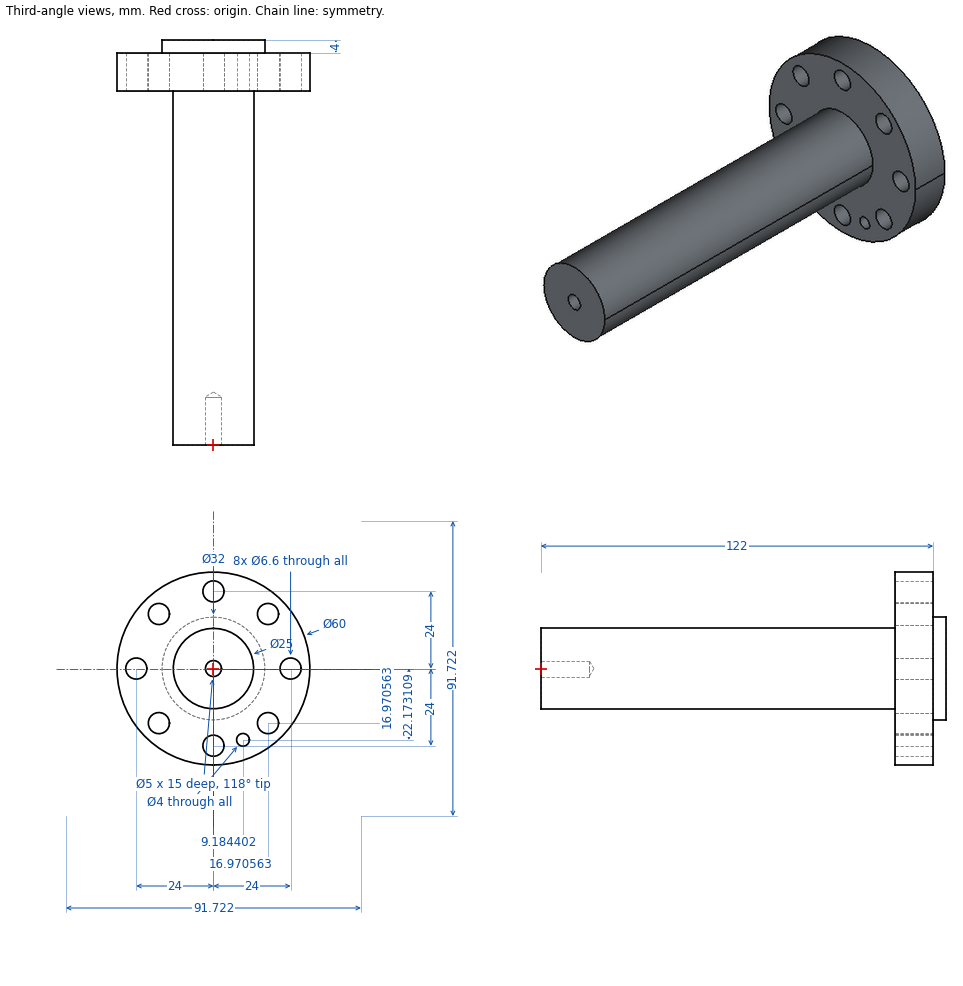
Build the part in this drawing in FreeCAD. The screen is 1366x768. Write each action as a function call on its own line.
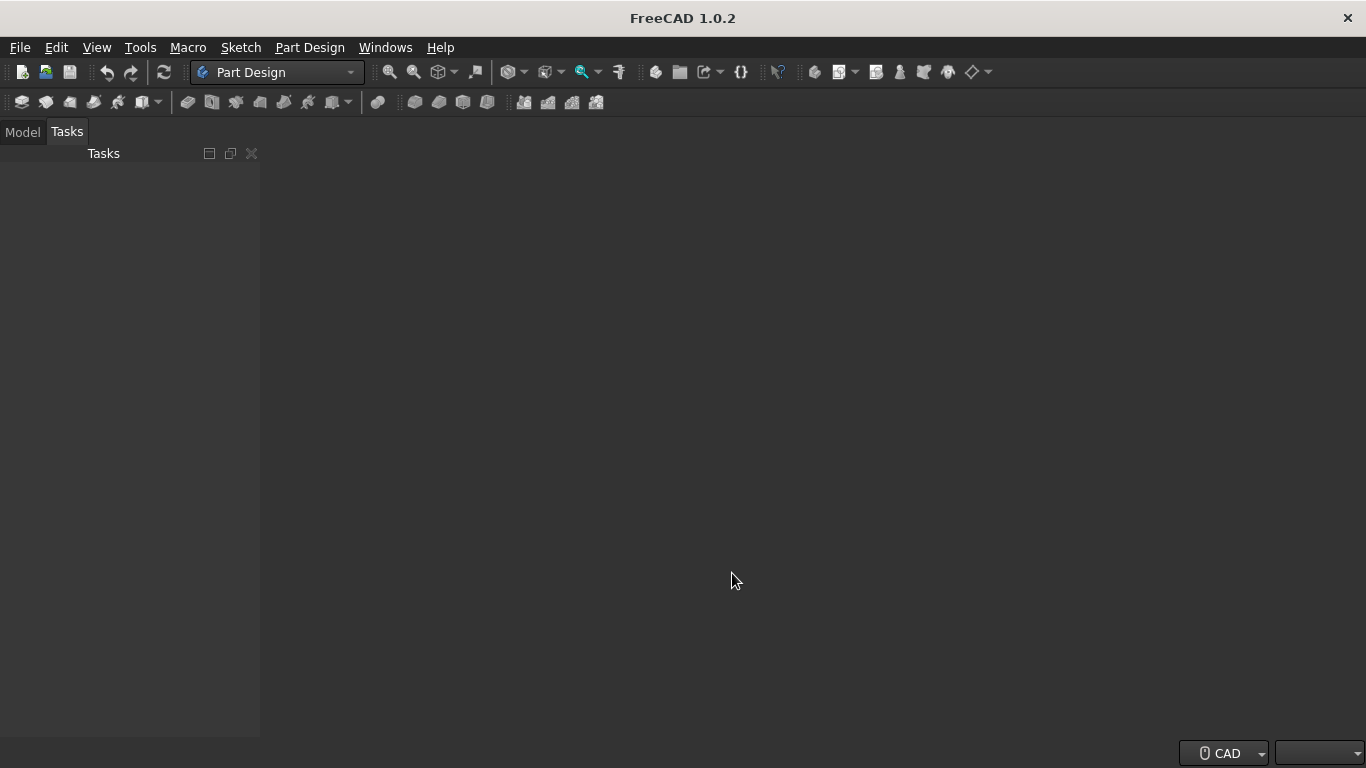
click(22, 72)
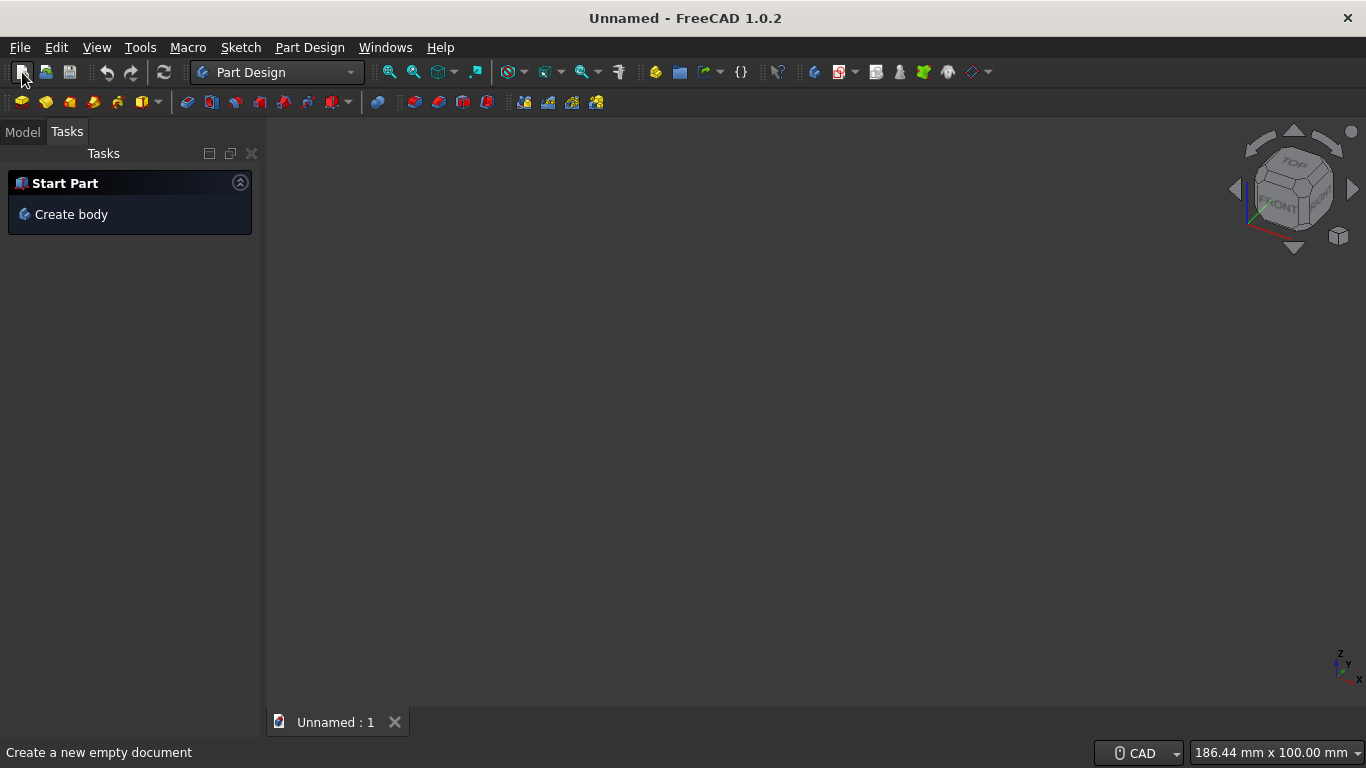
click(840, 72)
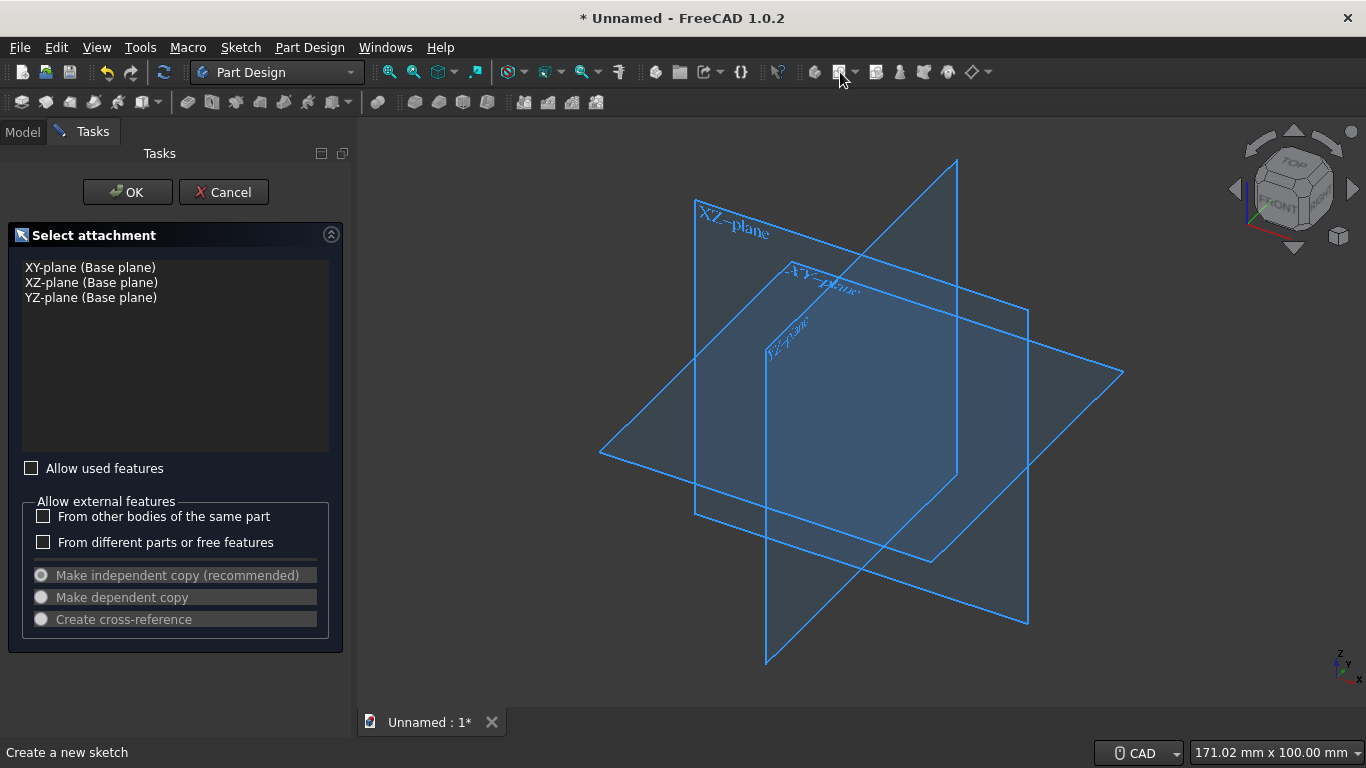
click(82, 282)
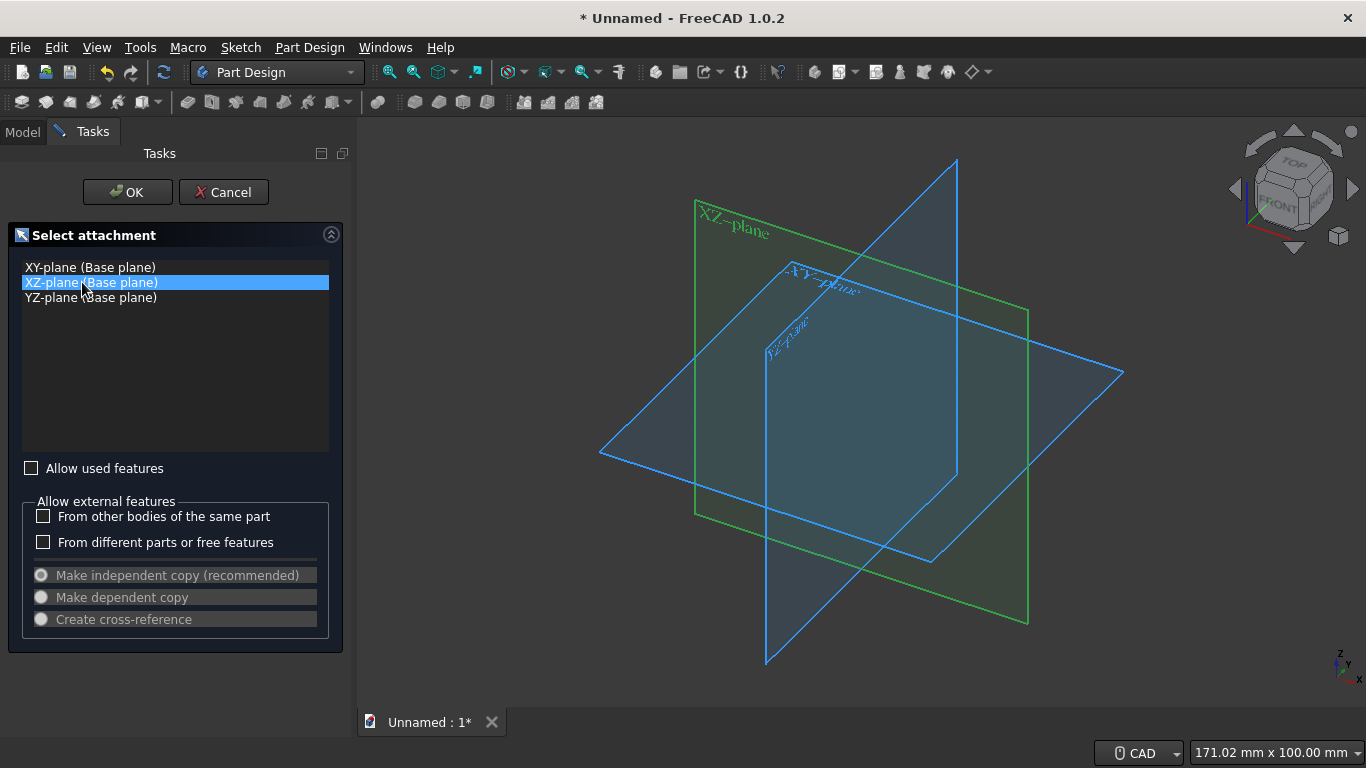
click(128, 192)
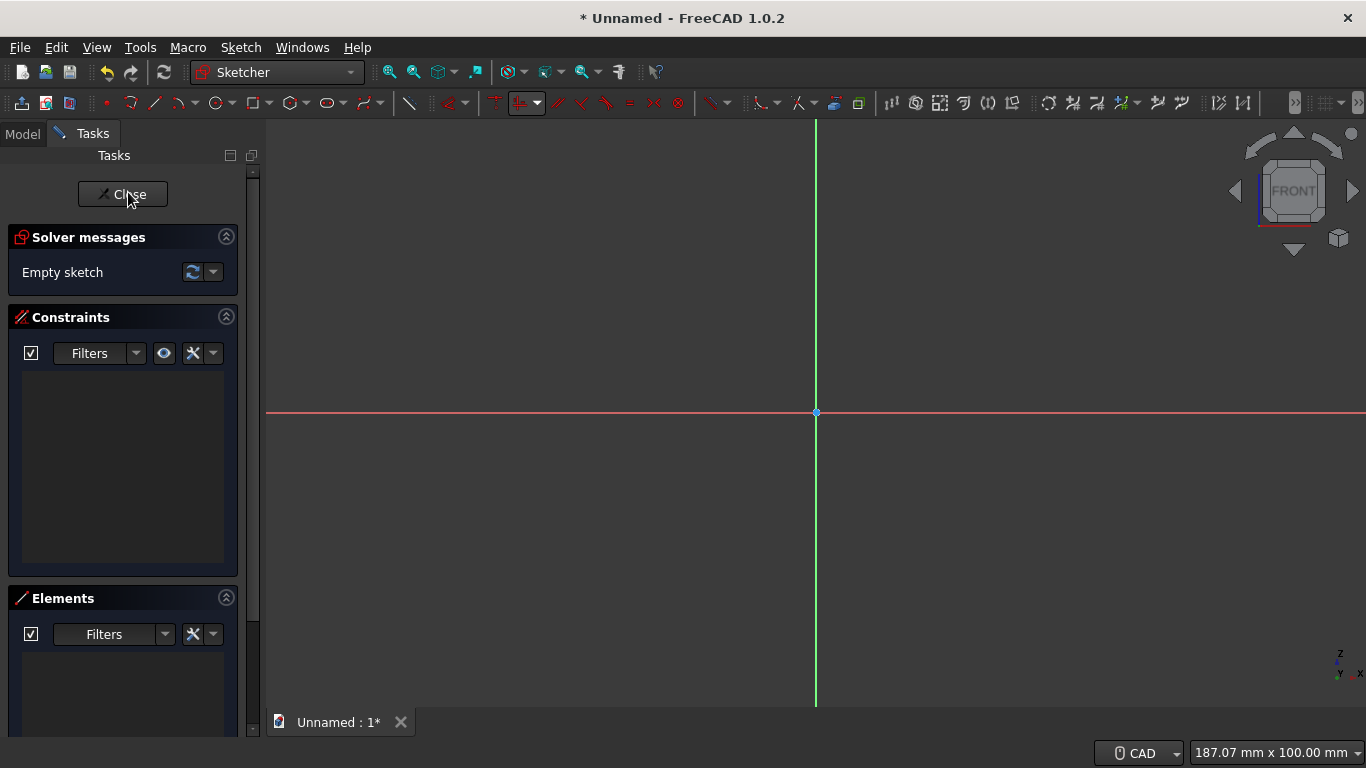
key(g)
key(c)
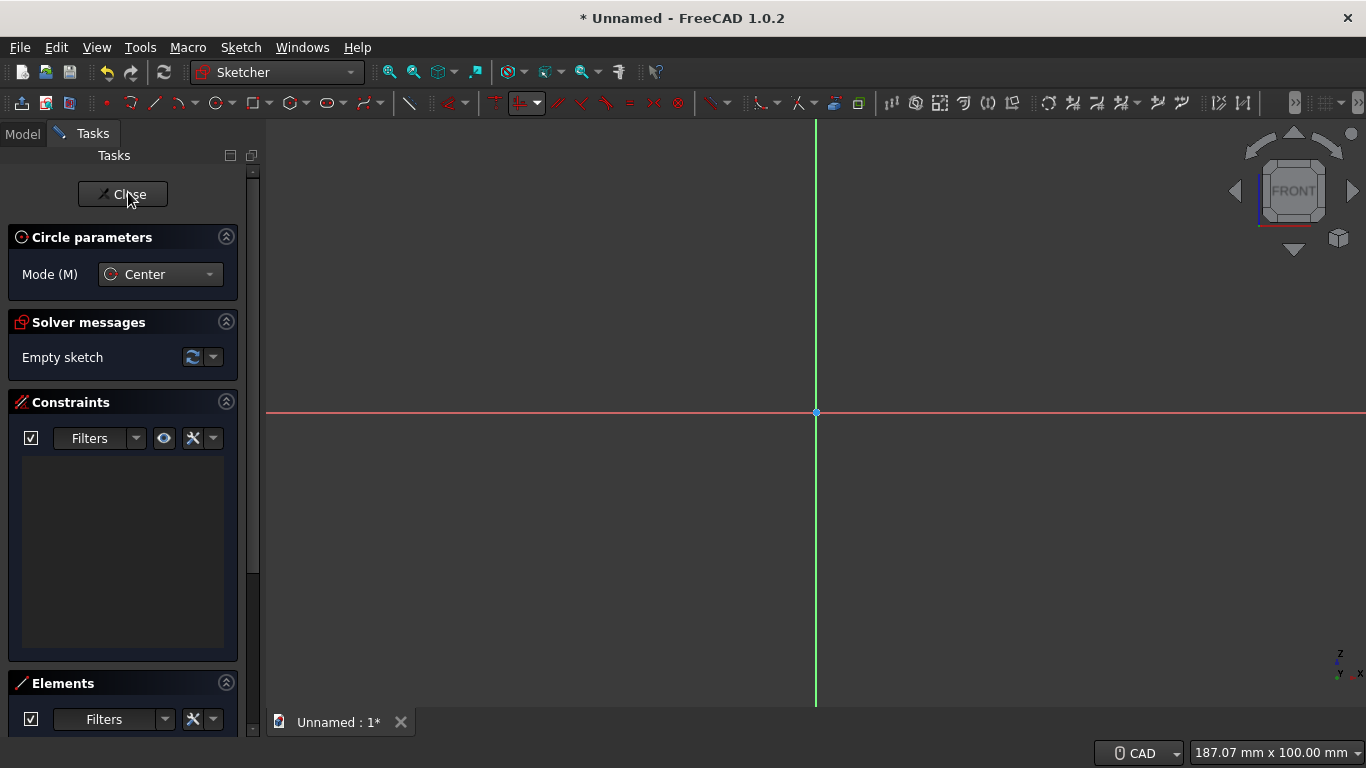
click(816, 413)
click(941, 288)
key(Escape)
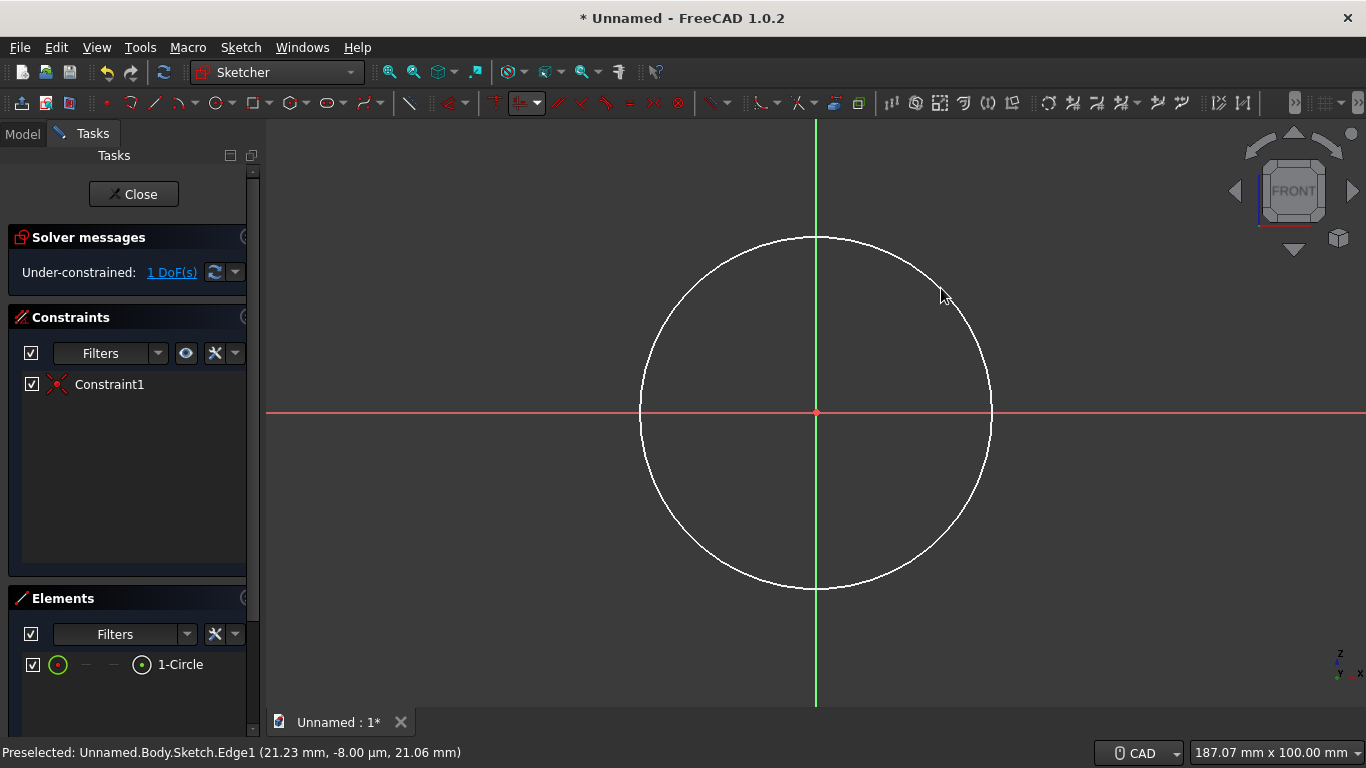
click(940, 288)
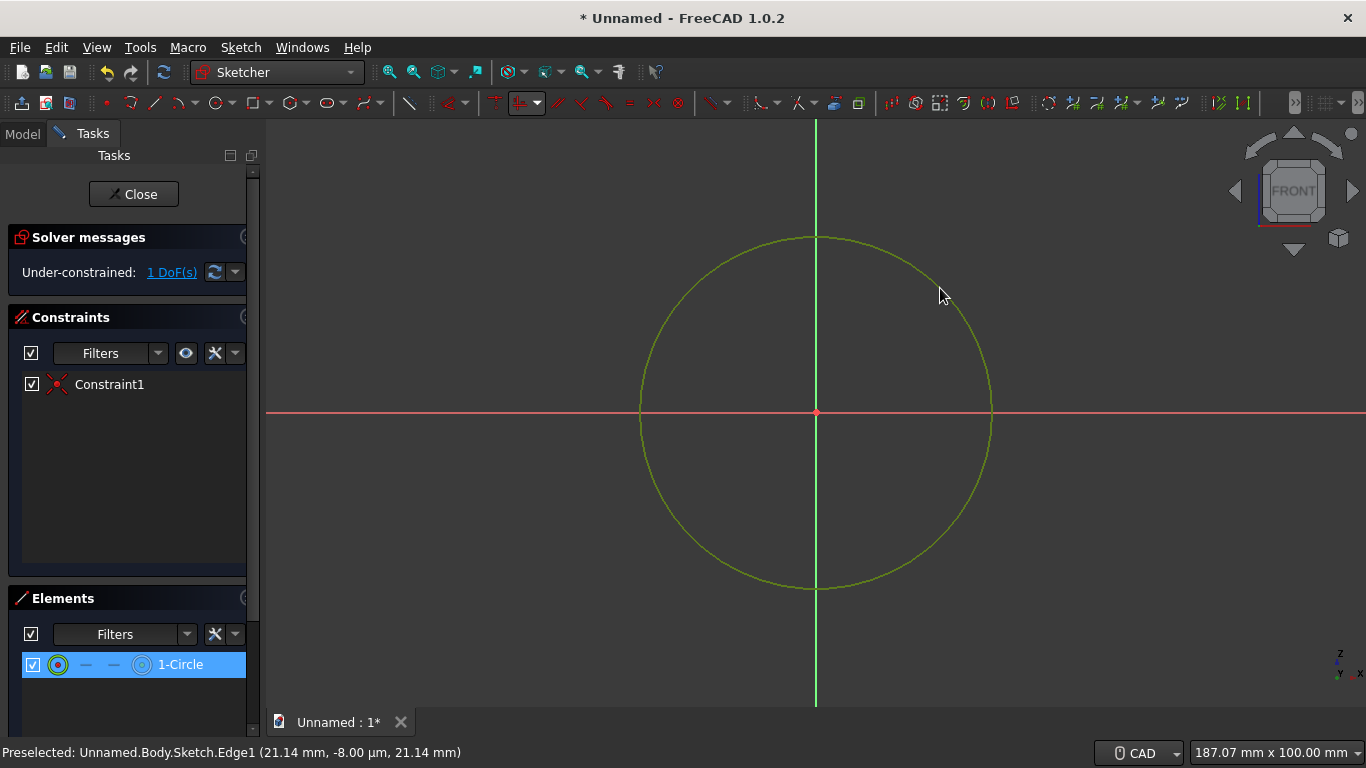
click(468, 104)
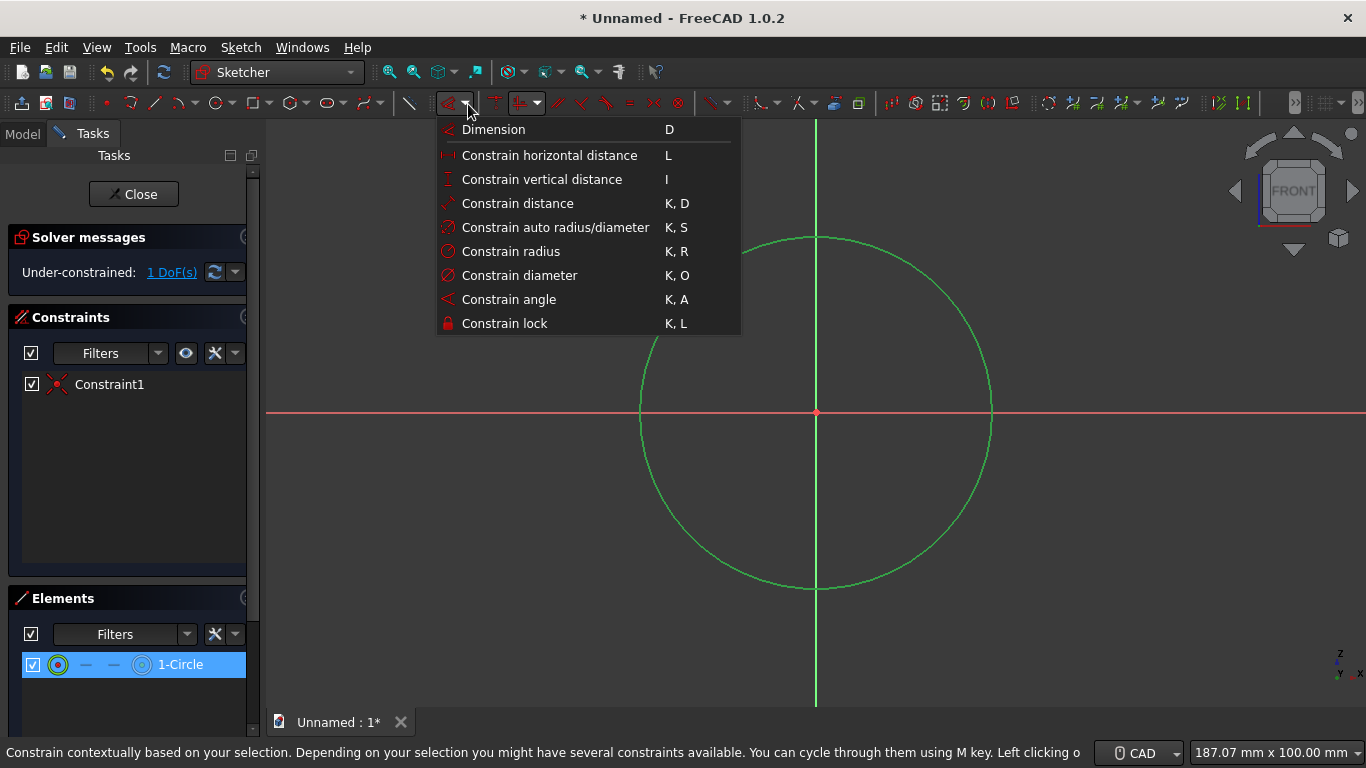
click(589, 275)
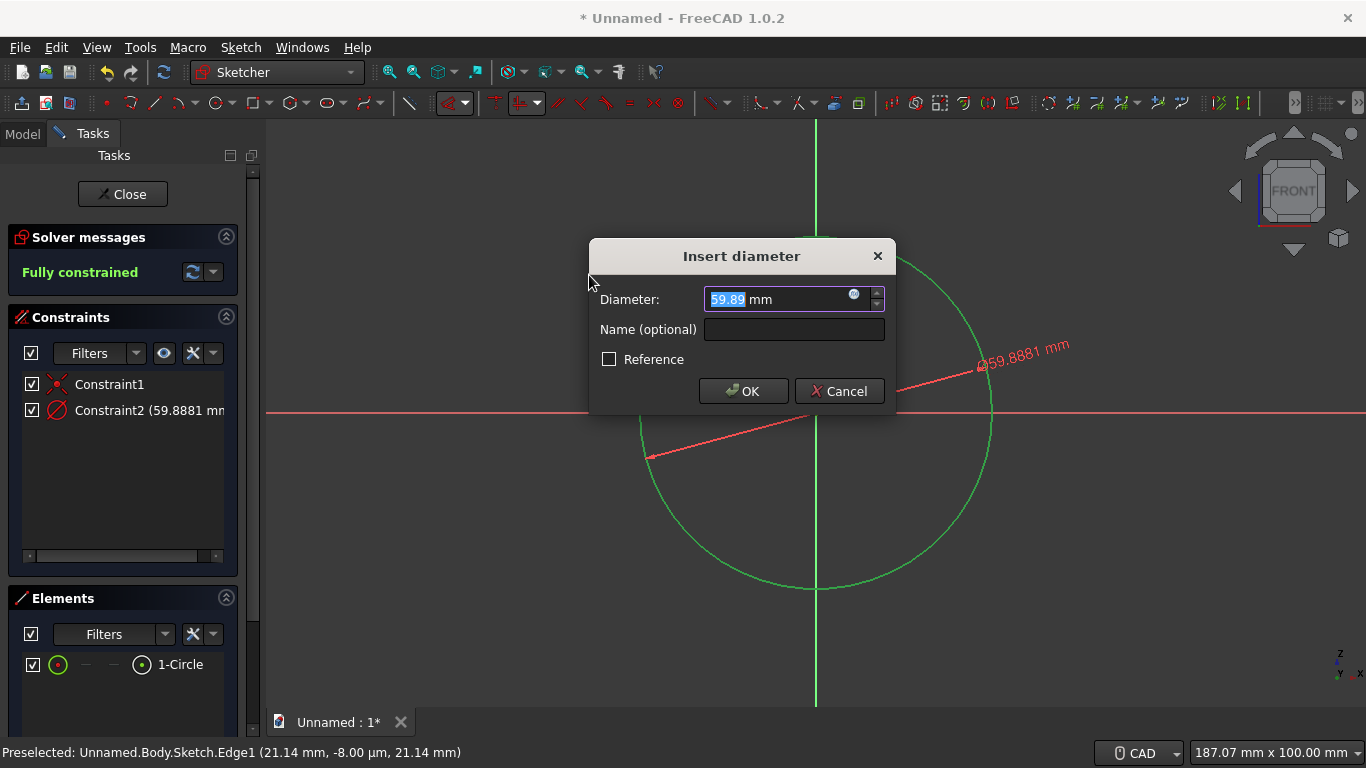
text(60)
key(Return)